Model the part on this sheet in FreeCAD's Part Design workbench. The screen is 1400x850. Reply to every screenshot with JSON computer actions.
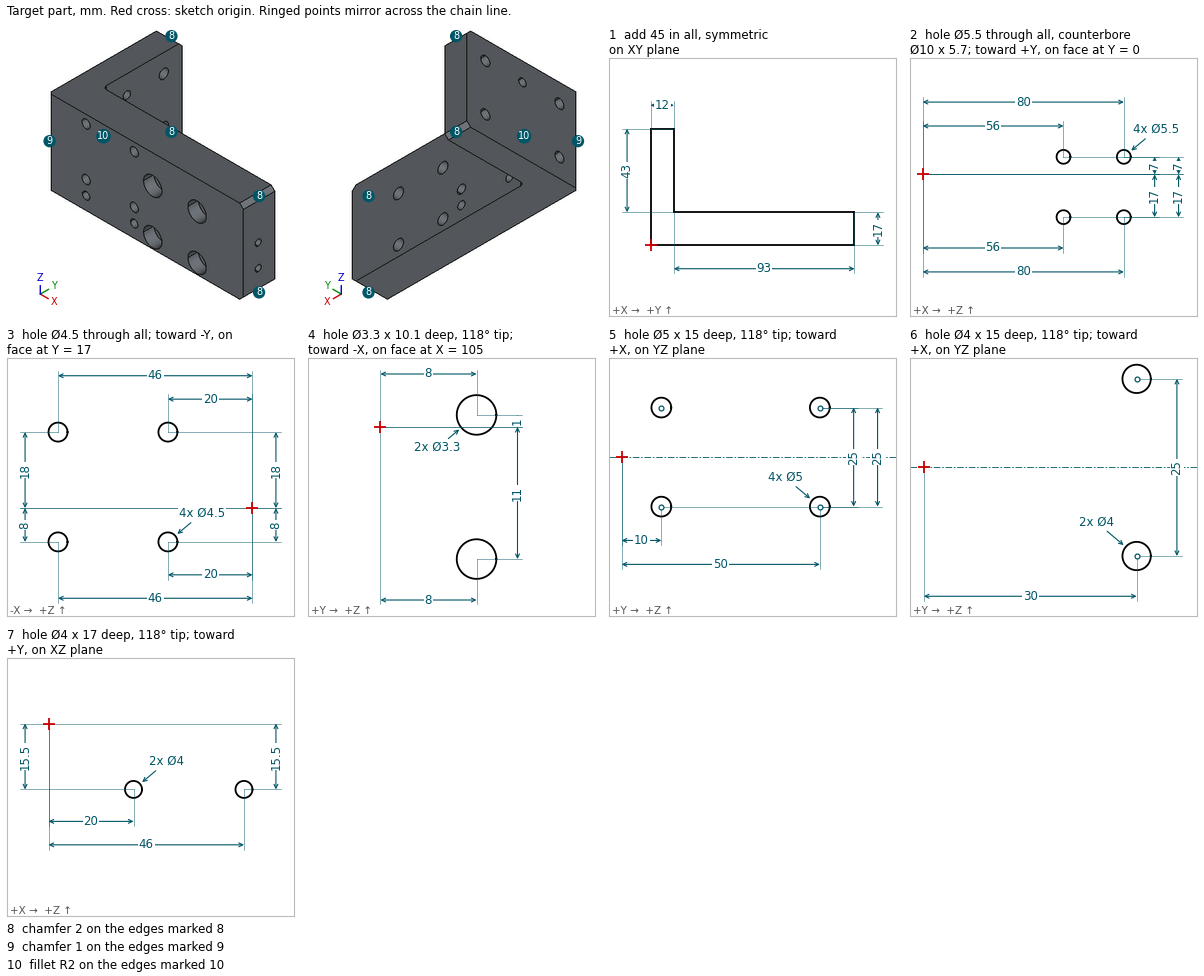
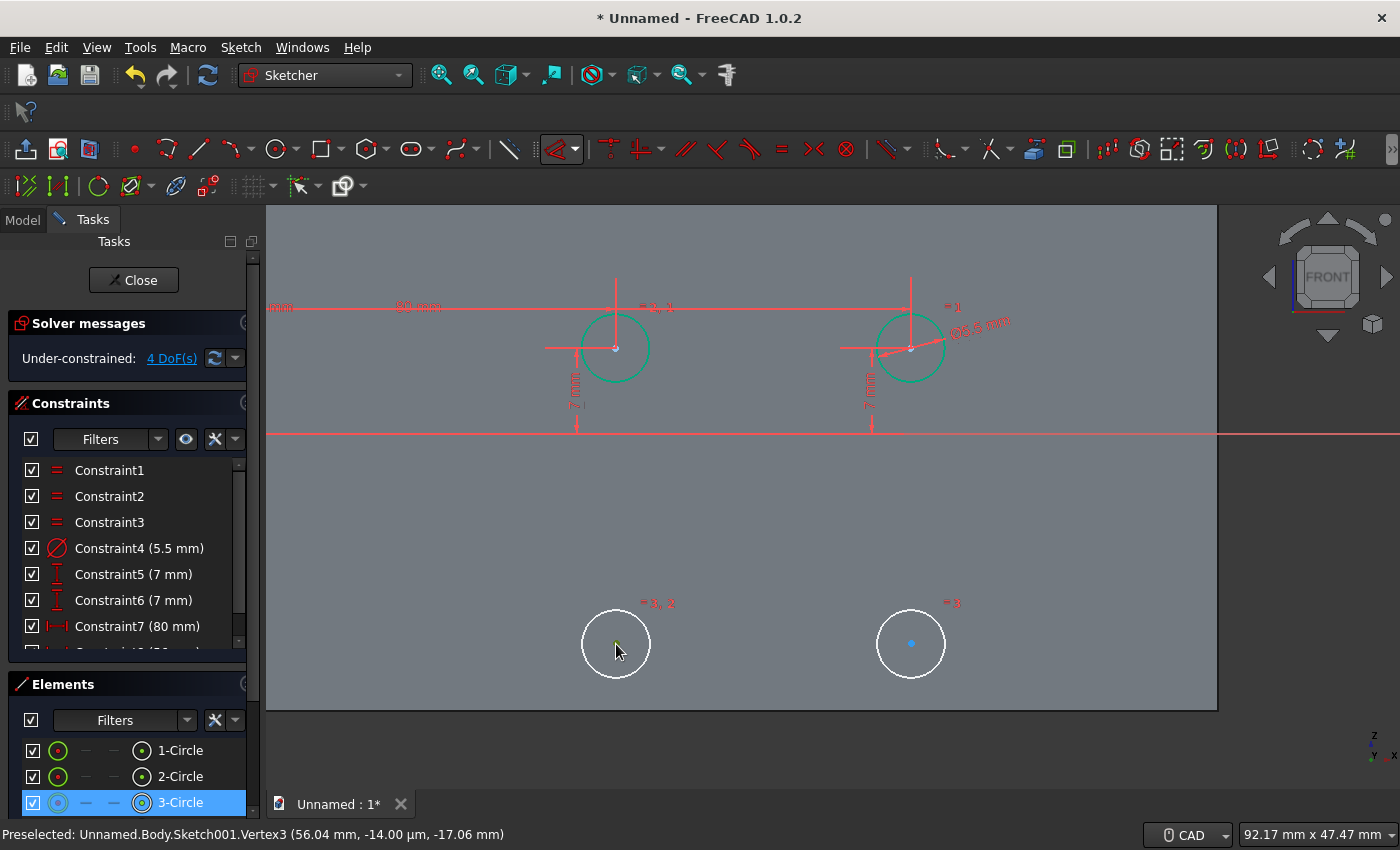
{"action": "key", "text": "l"}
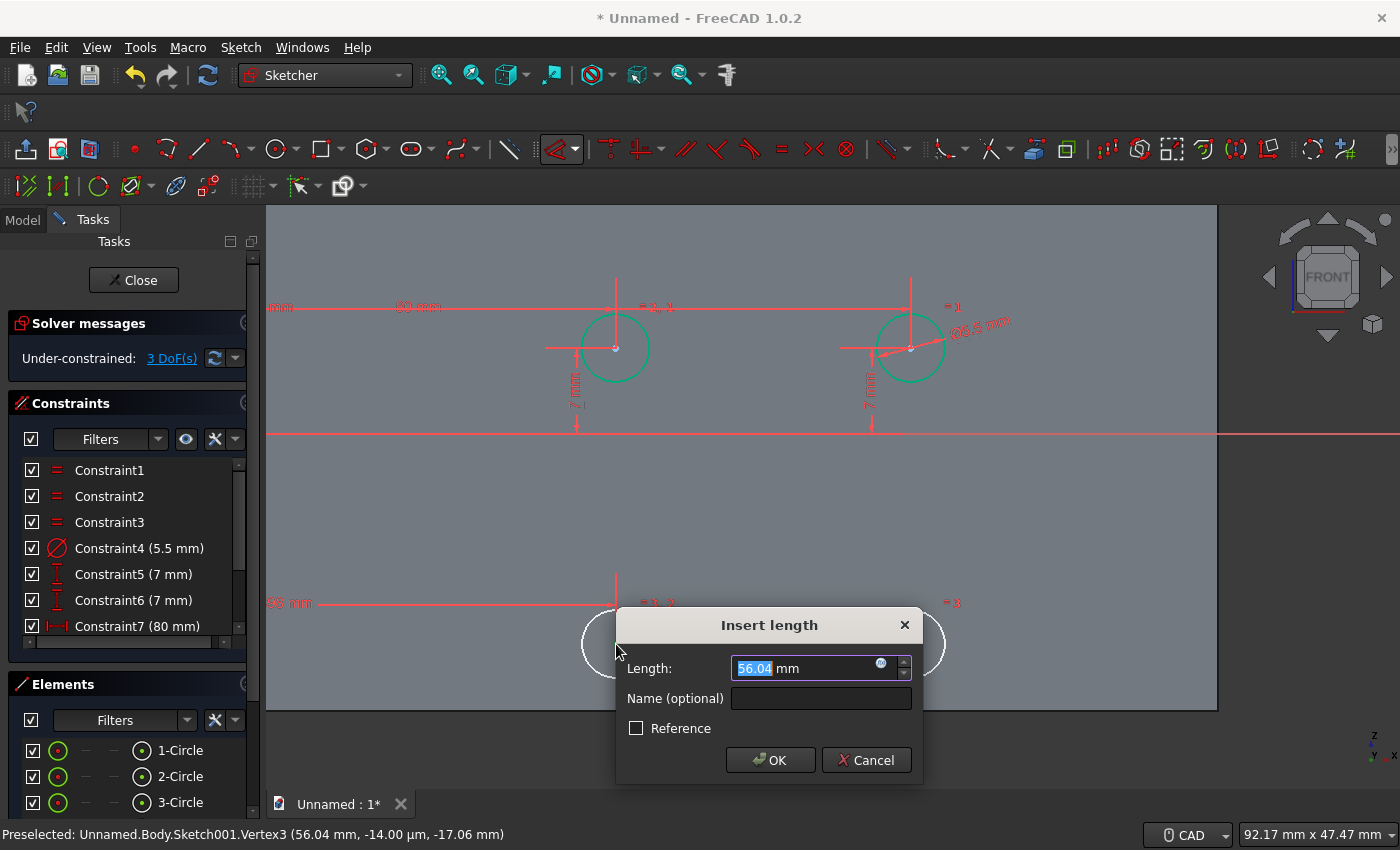
{"action": "type", "text": "56"}
{"action": "key", "text": "Return"}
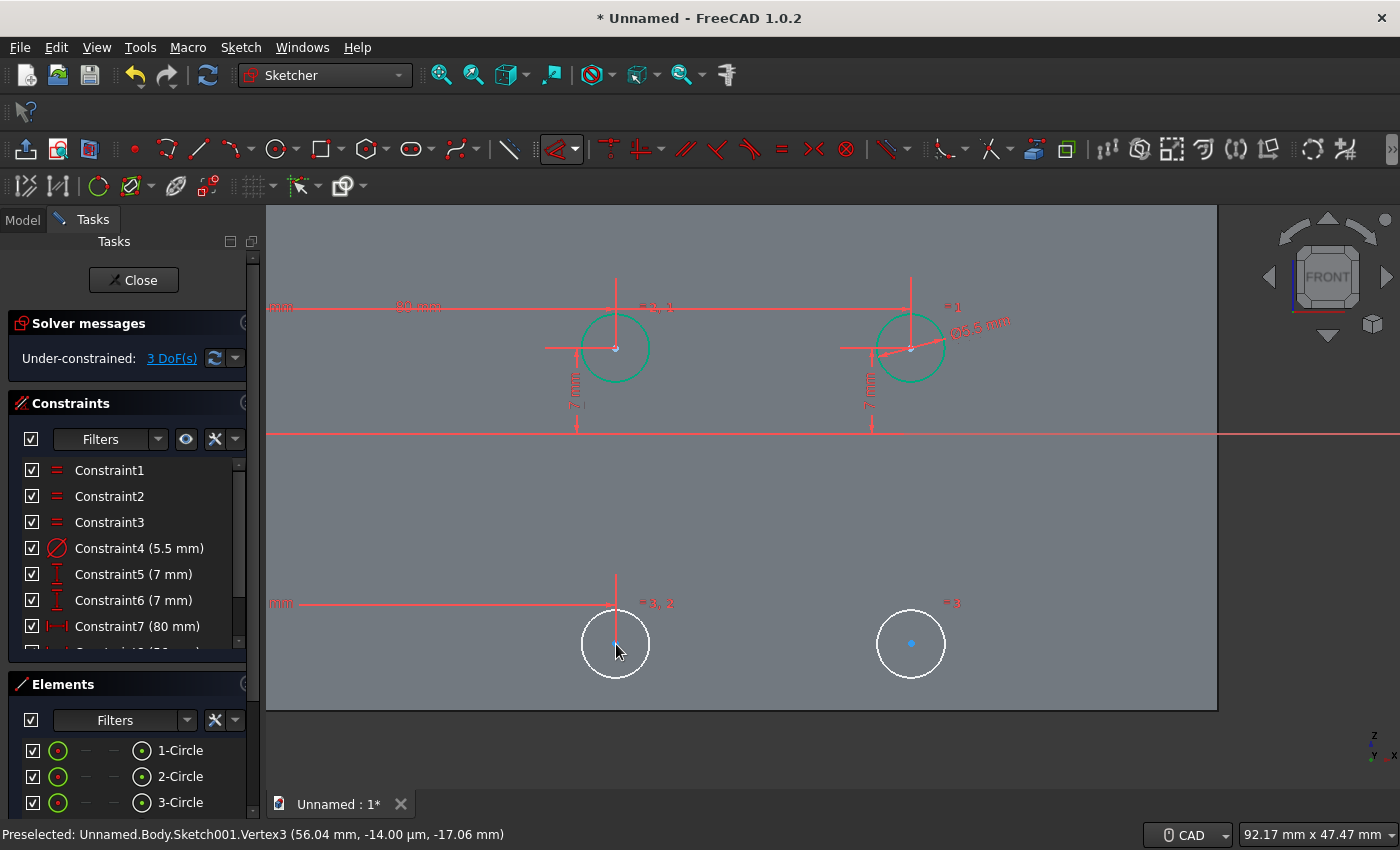
{"action": "left_click", "coordinate": [616, 644]}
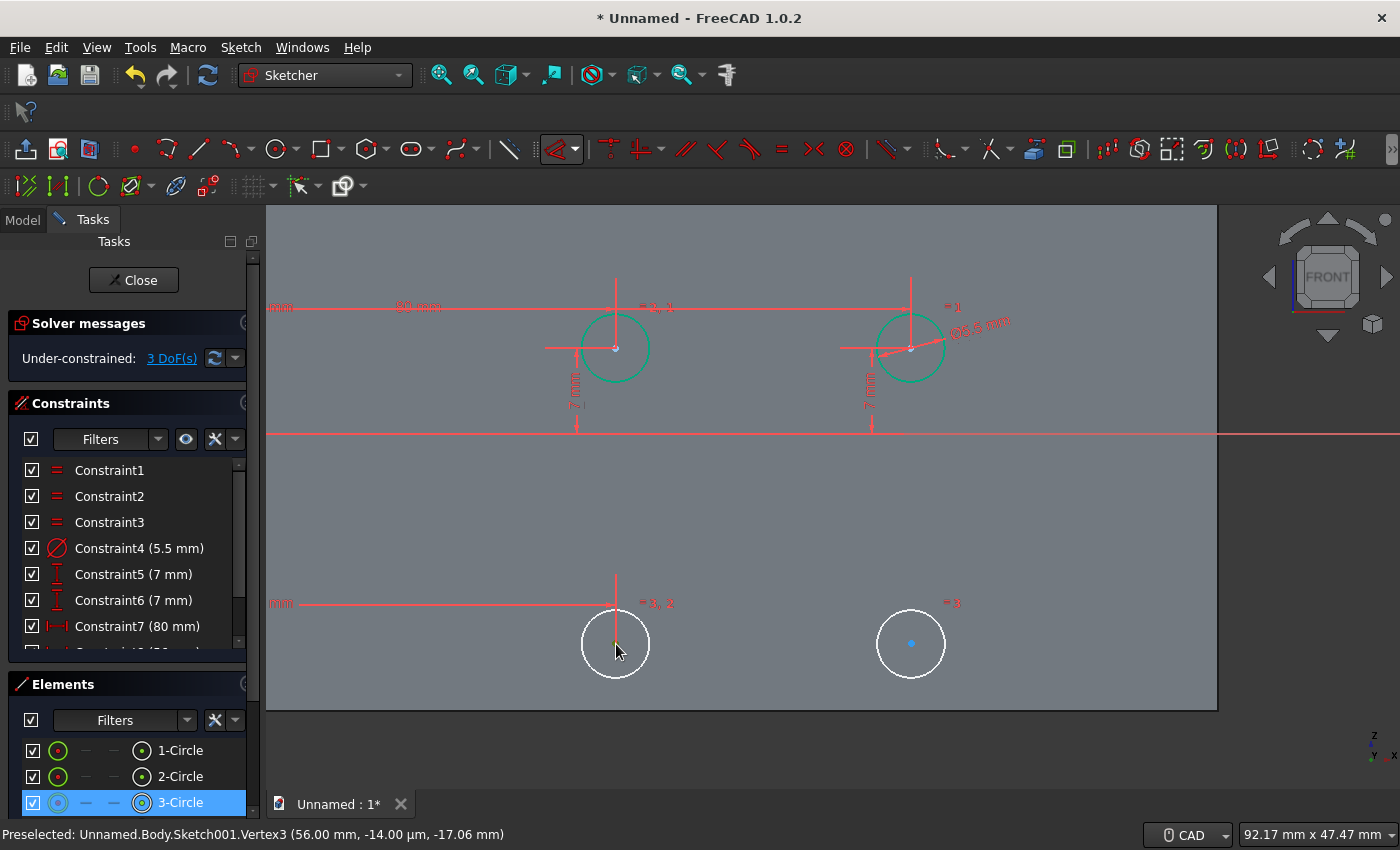
{"action": "left_click", "coordinate": [578, 150]}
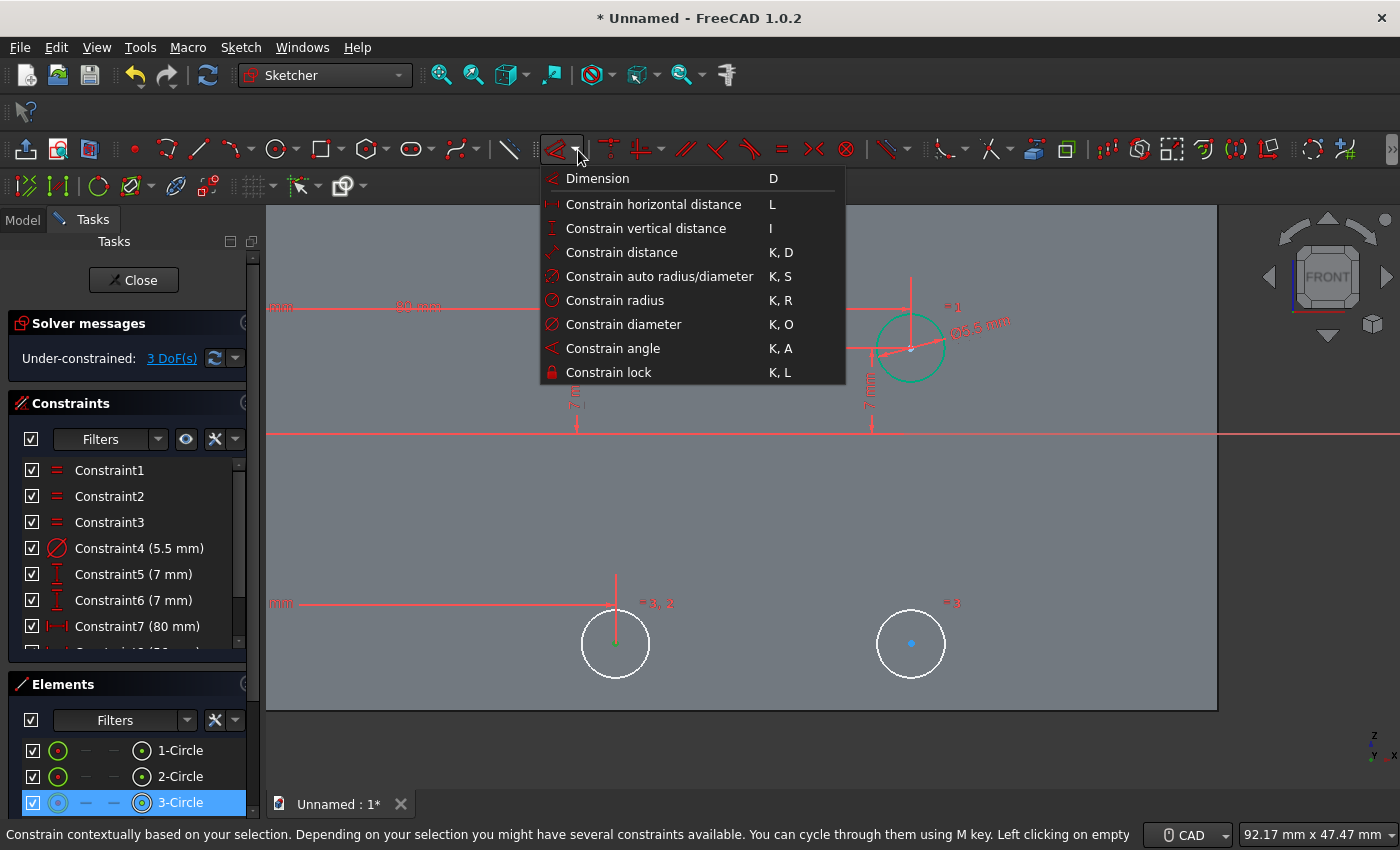
{"action": "left_click", "coordinate": [693, 228]}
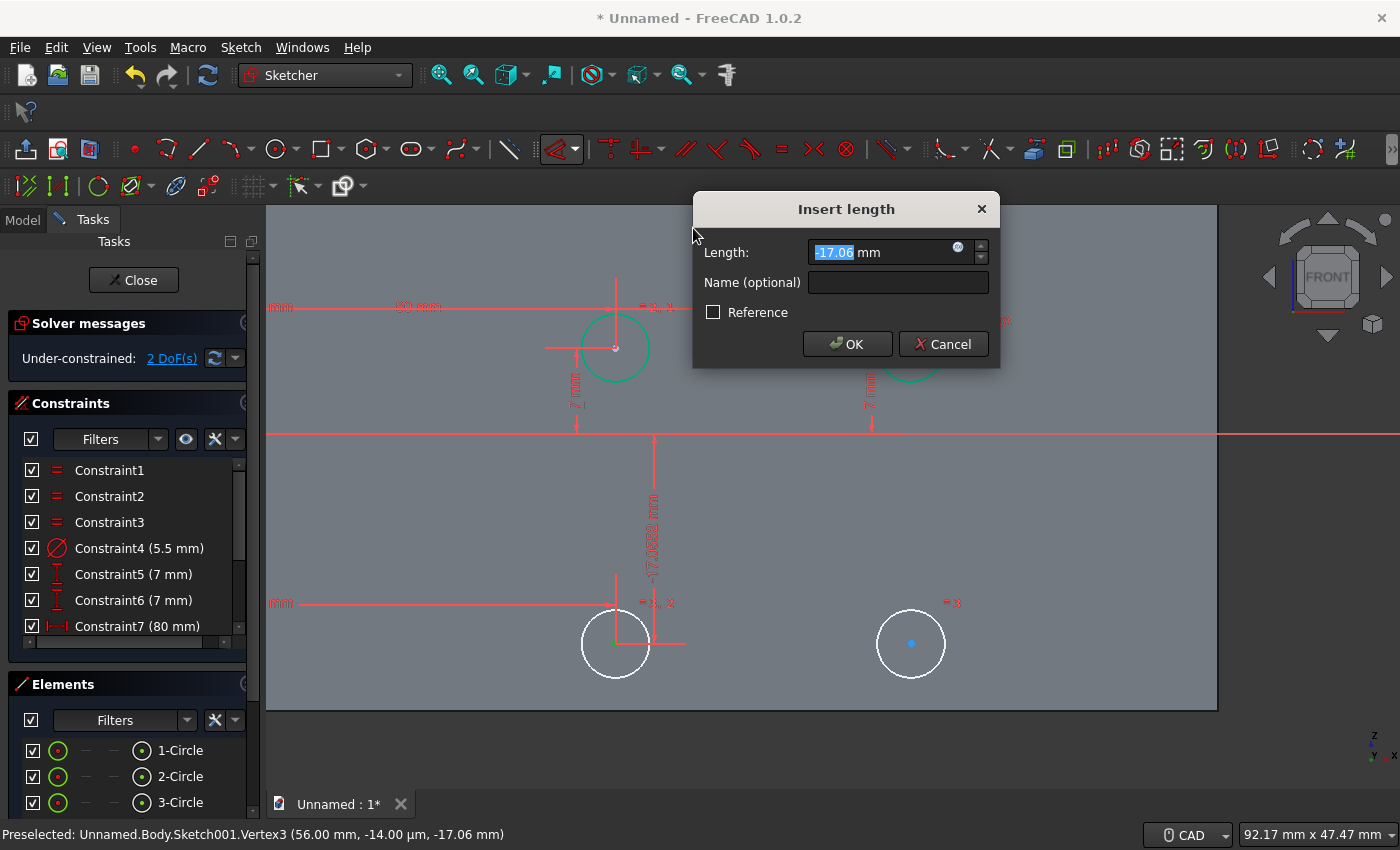
{"action": "type", "text": "-17"}
{"action": "key", "text": "Return"}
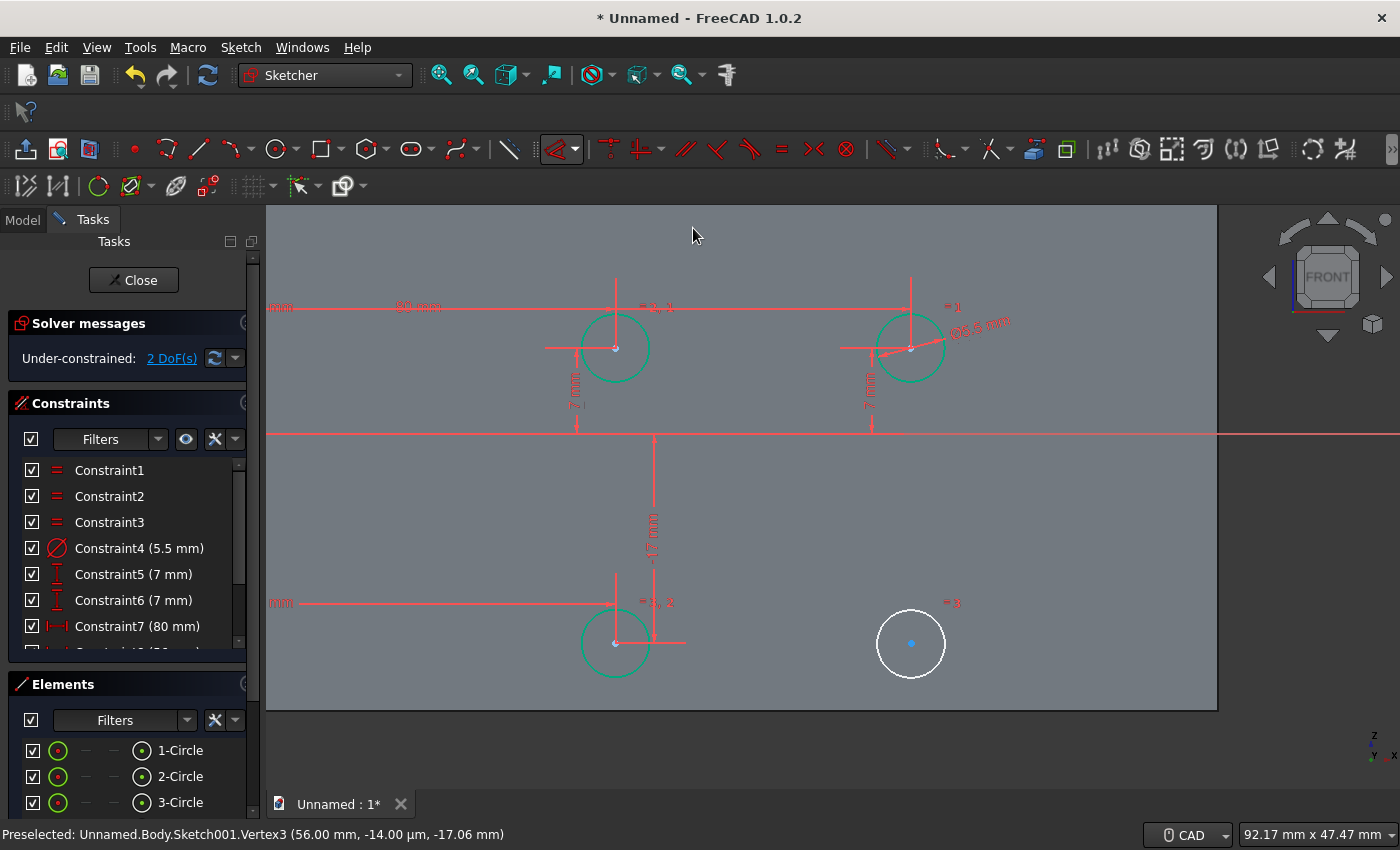
{"action": "left_click", "coordinate": [911, 644]}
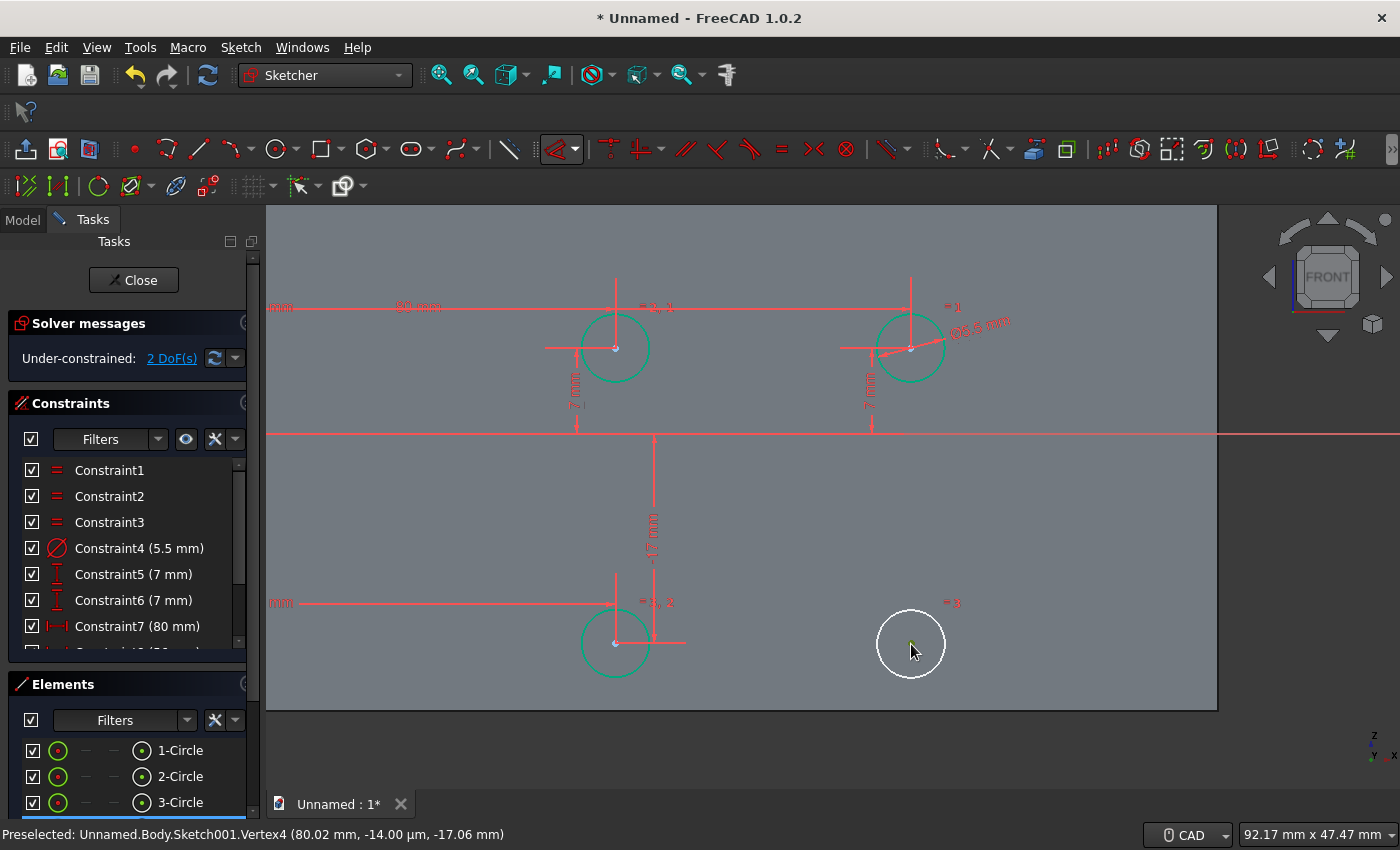
{"action": "key", "text": "l"}